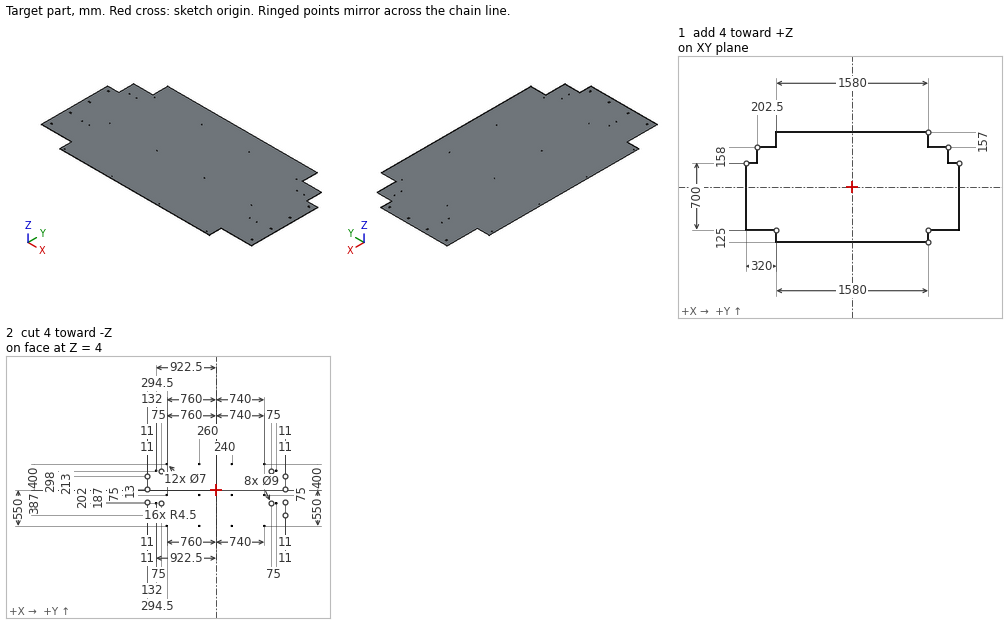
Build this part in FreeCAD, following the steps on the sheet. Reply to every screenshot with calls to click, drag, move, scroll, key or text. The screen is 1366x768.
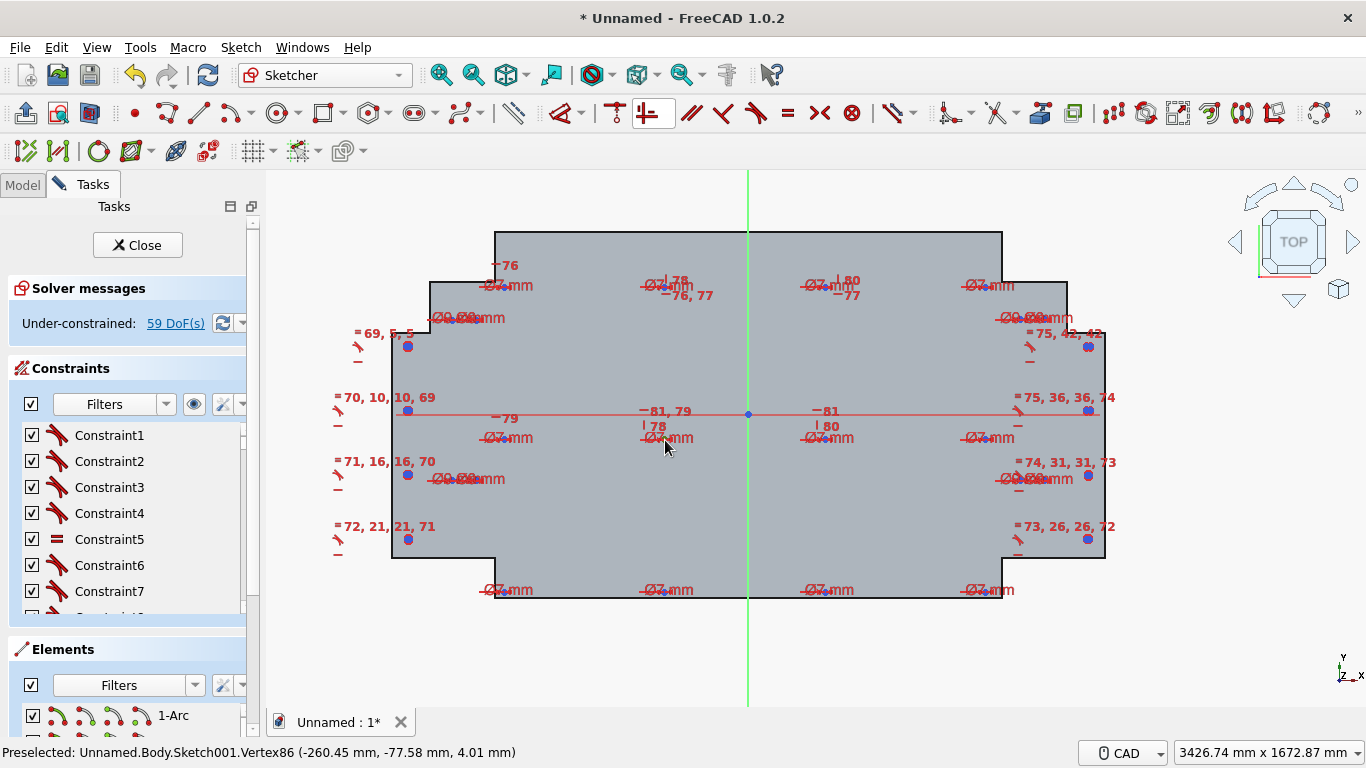
click(665, 592)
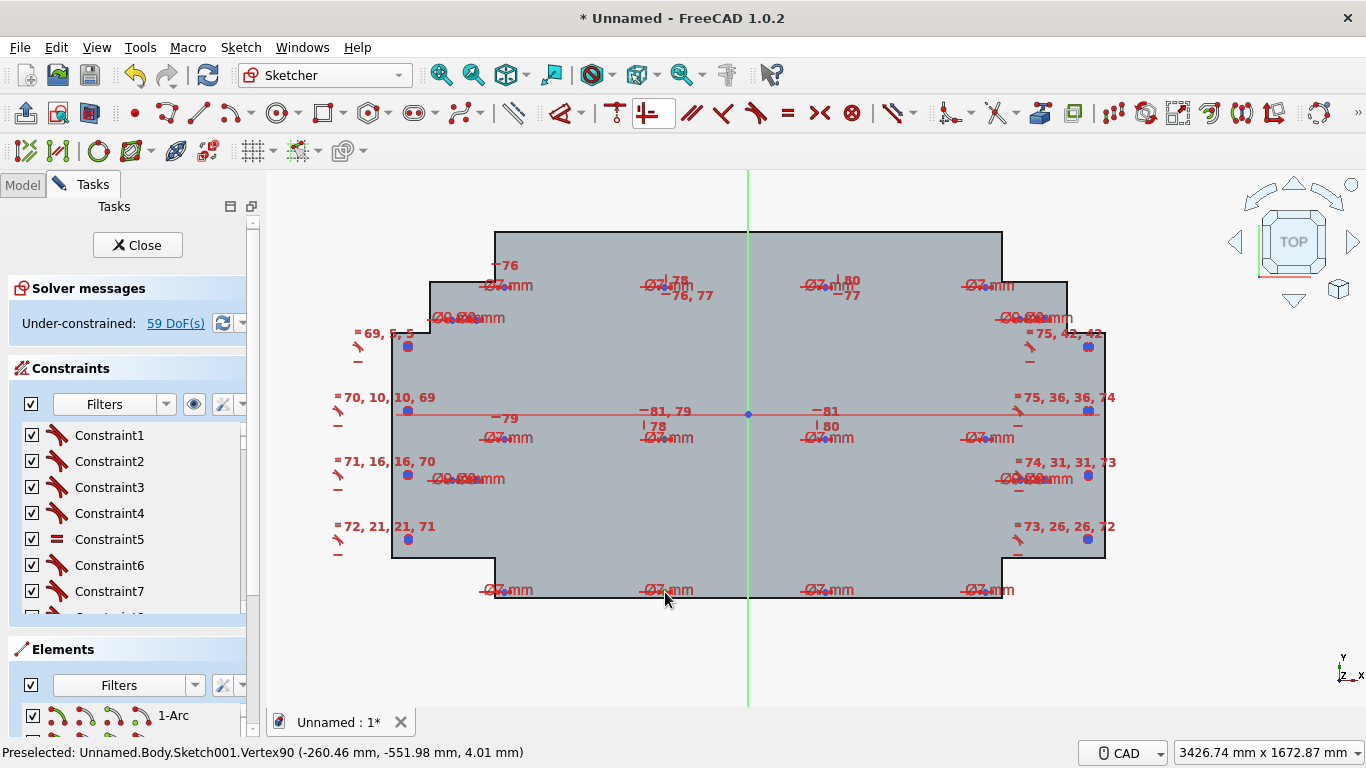
click(670, 114)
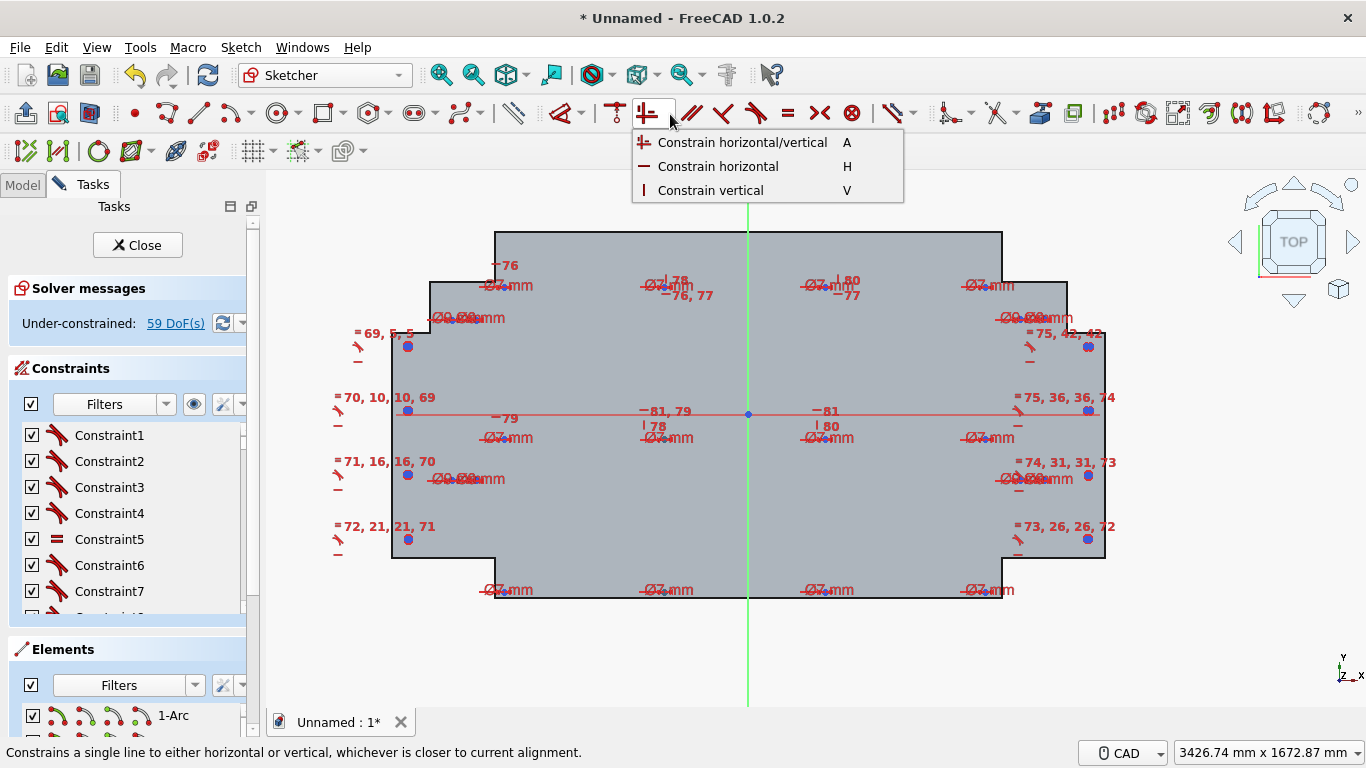
click(768, 190)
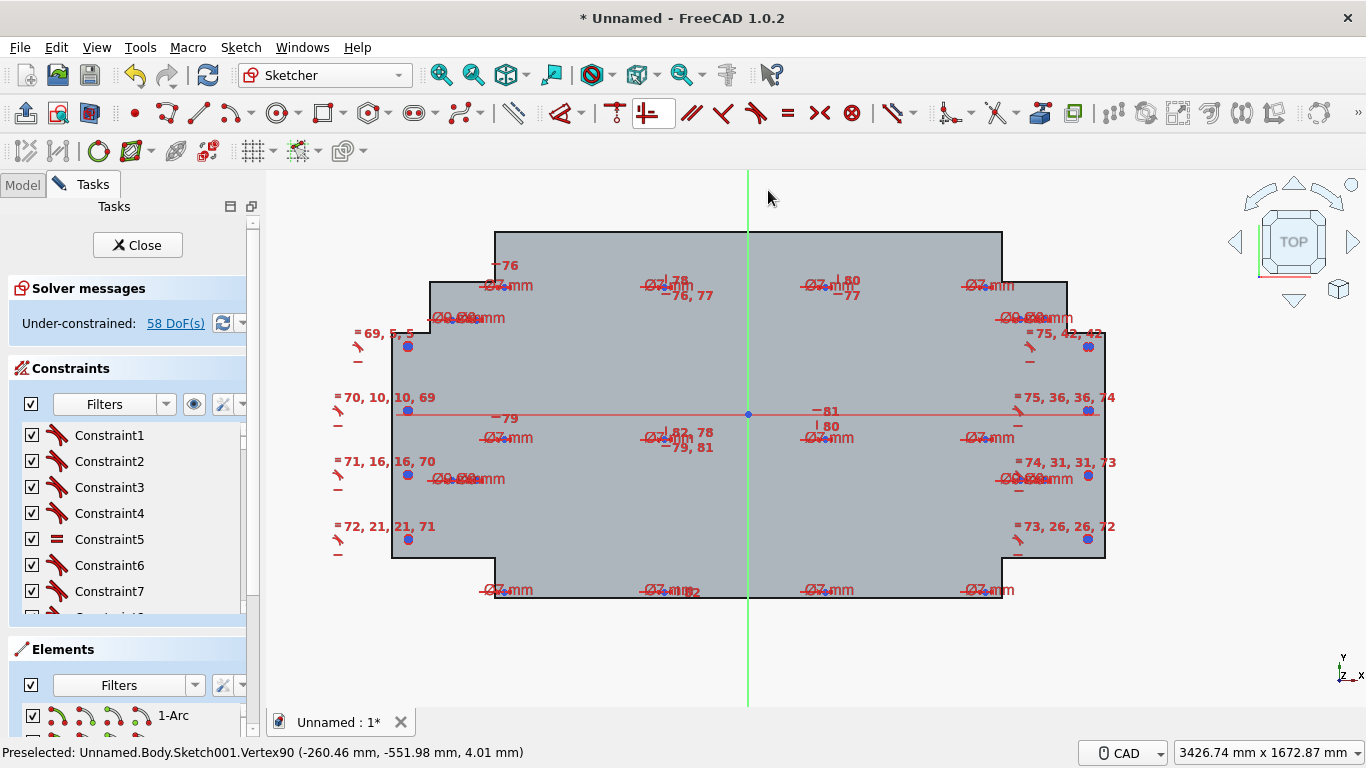
click(504, 592)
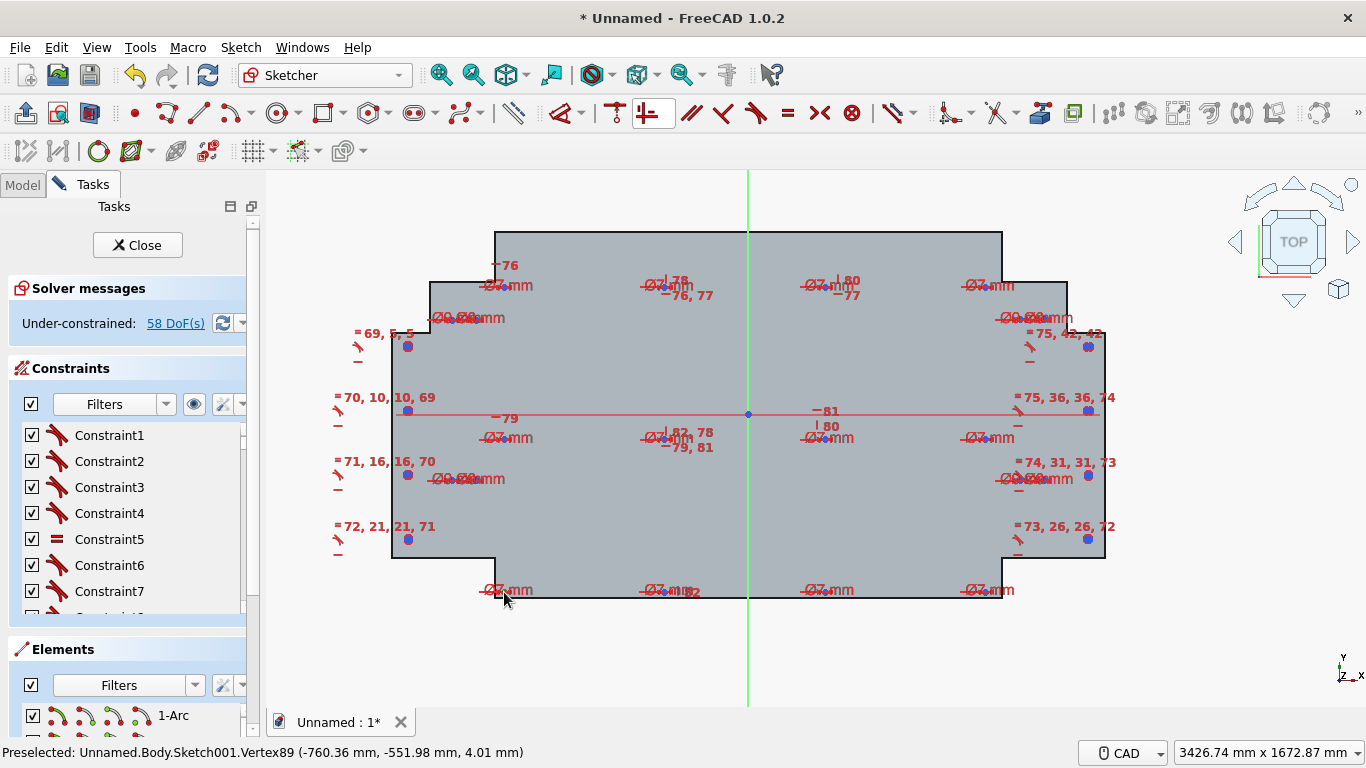
click(665, 592)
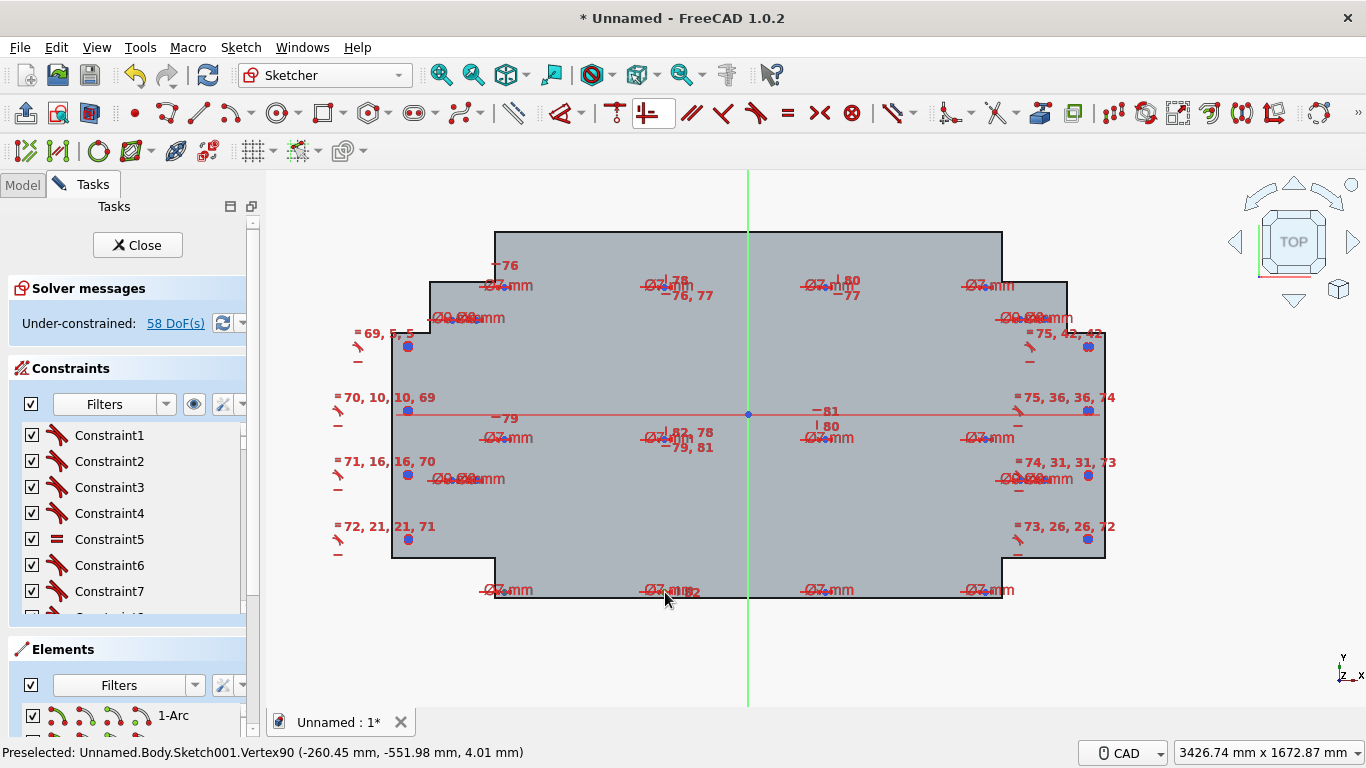
click(670, 114)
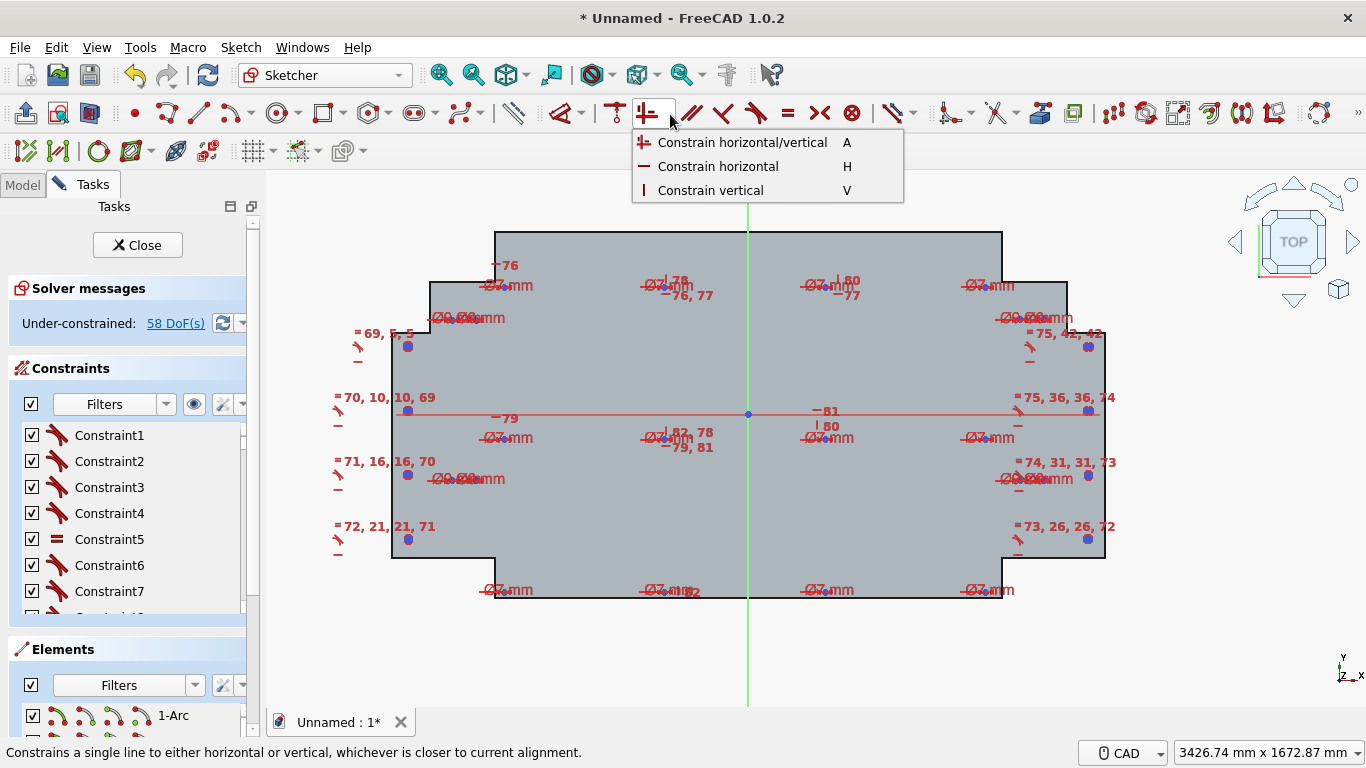
click(768, 166)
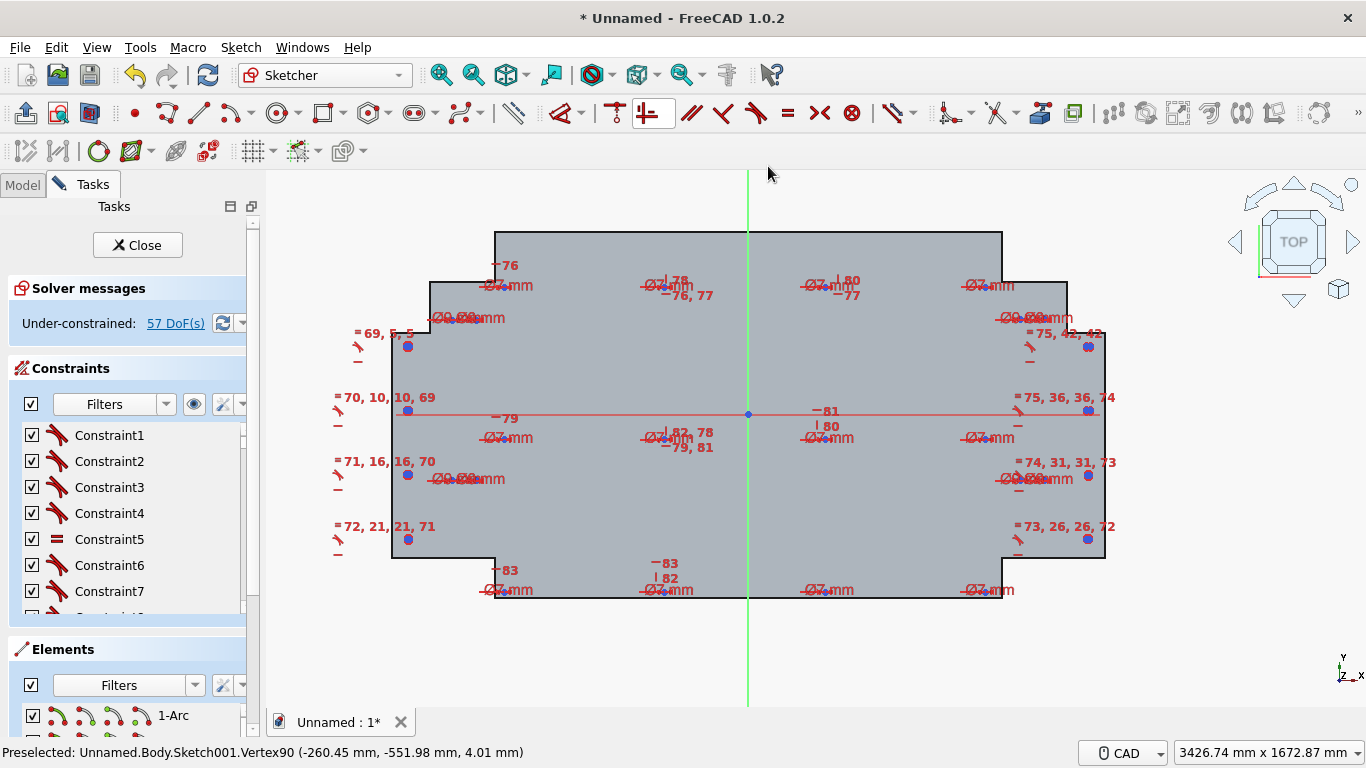
click(825, 440)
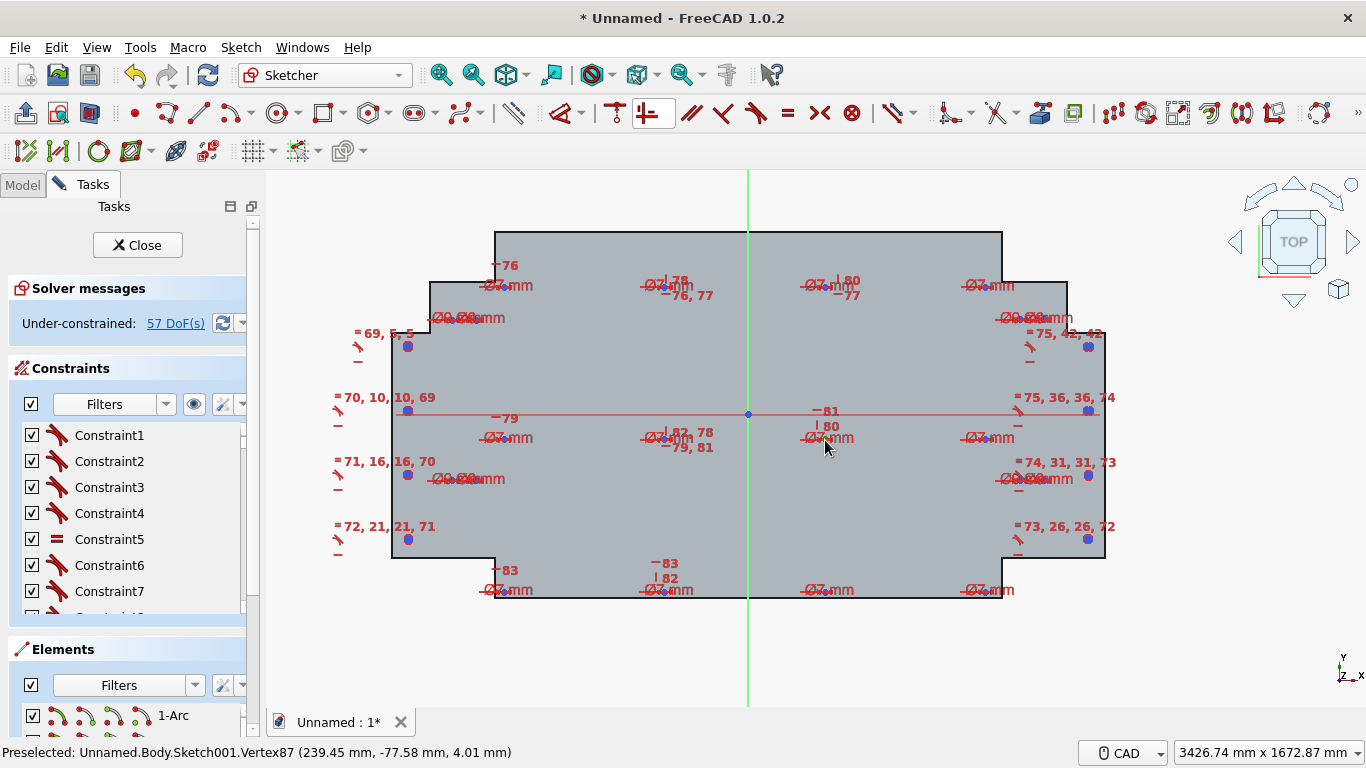
click(825, 592)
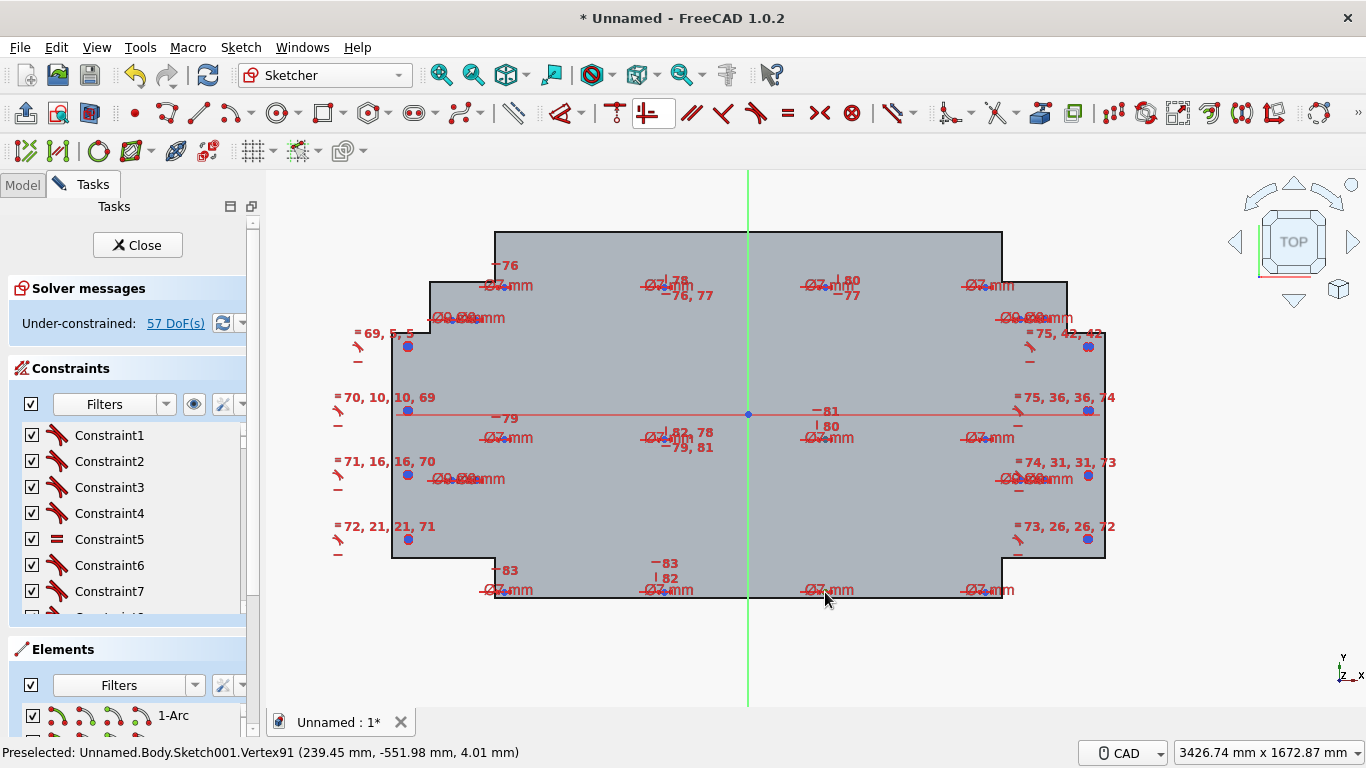
key(v)